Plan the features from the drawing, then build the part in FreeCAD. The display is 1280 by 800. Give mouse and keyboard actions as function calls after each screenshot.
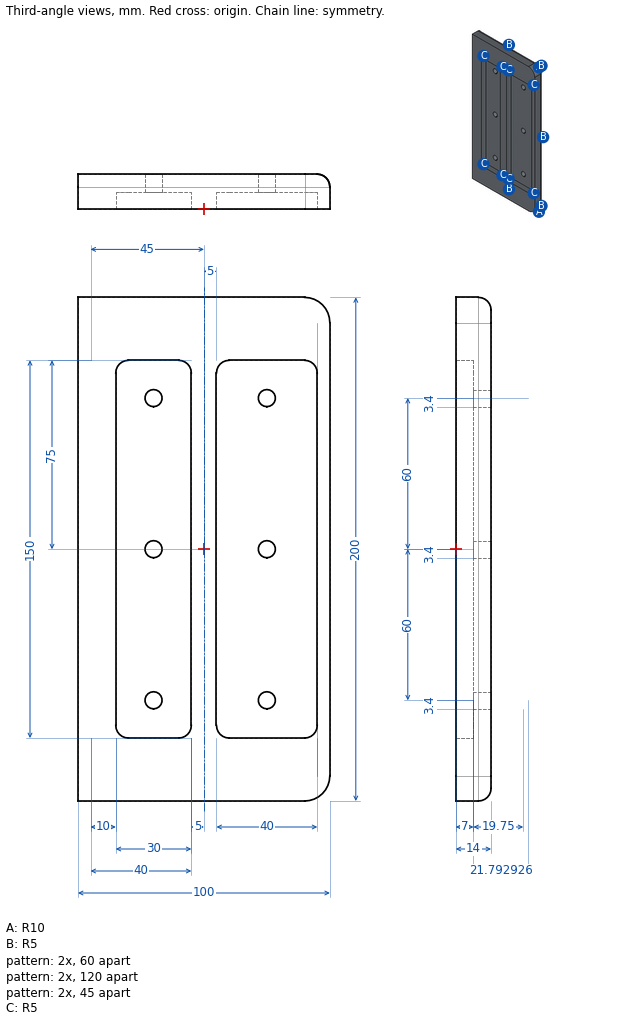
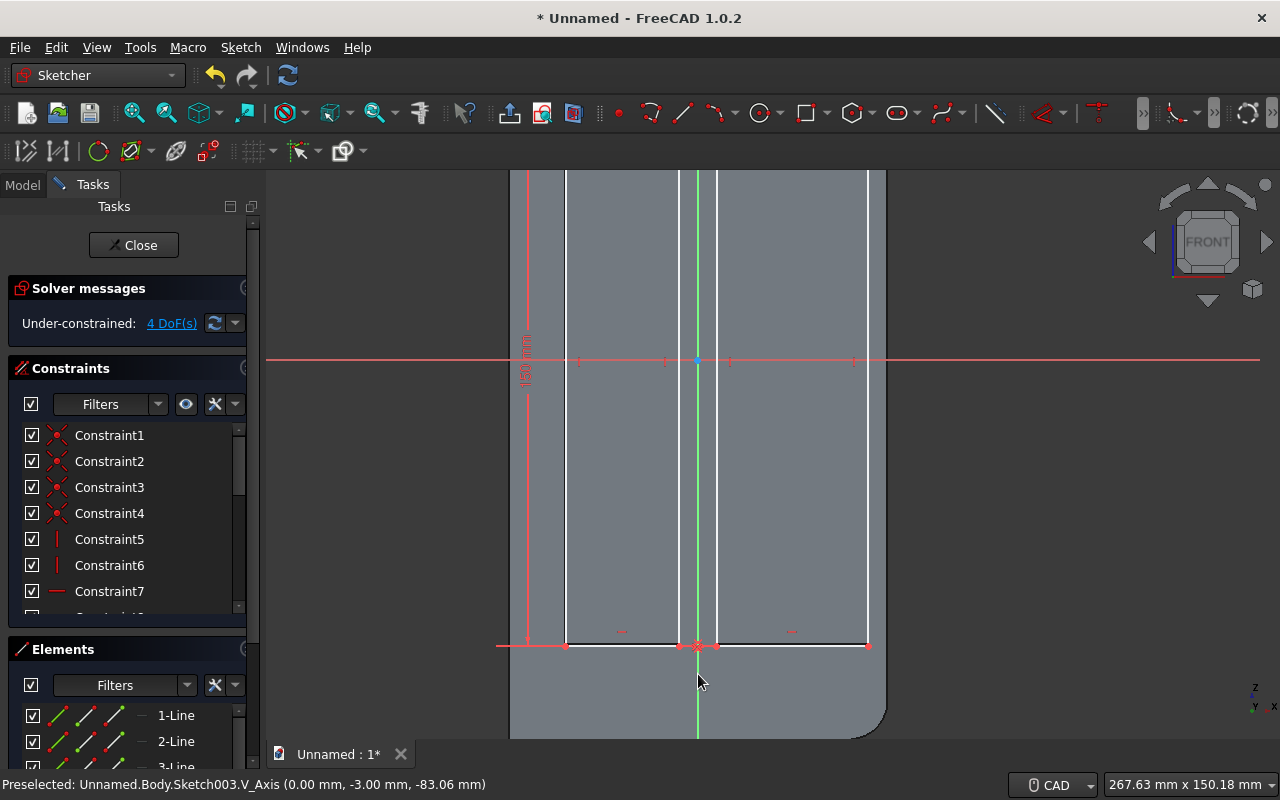
click(1042, 114)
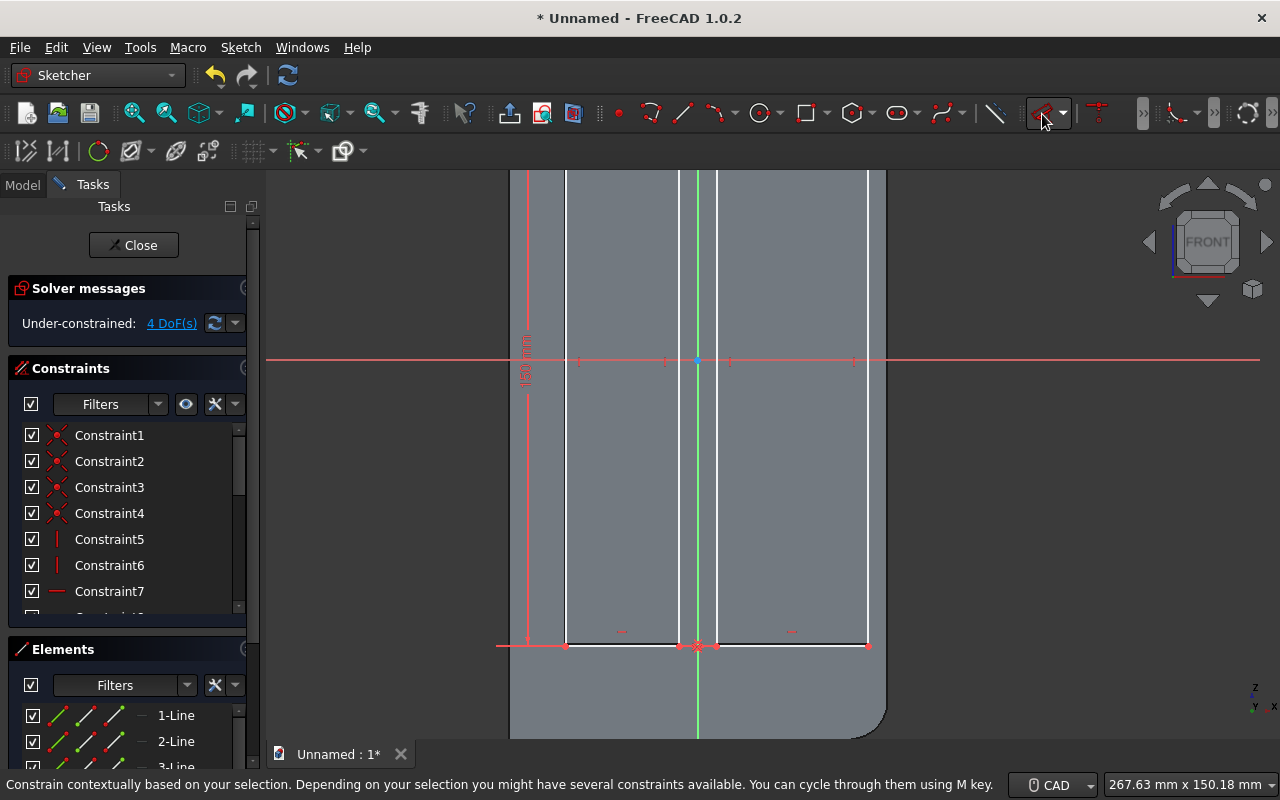
click(762, 646)
click(792, 680)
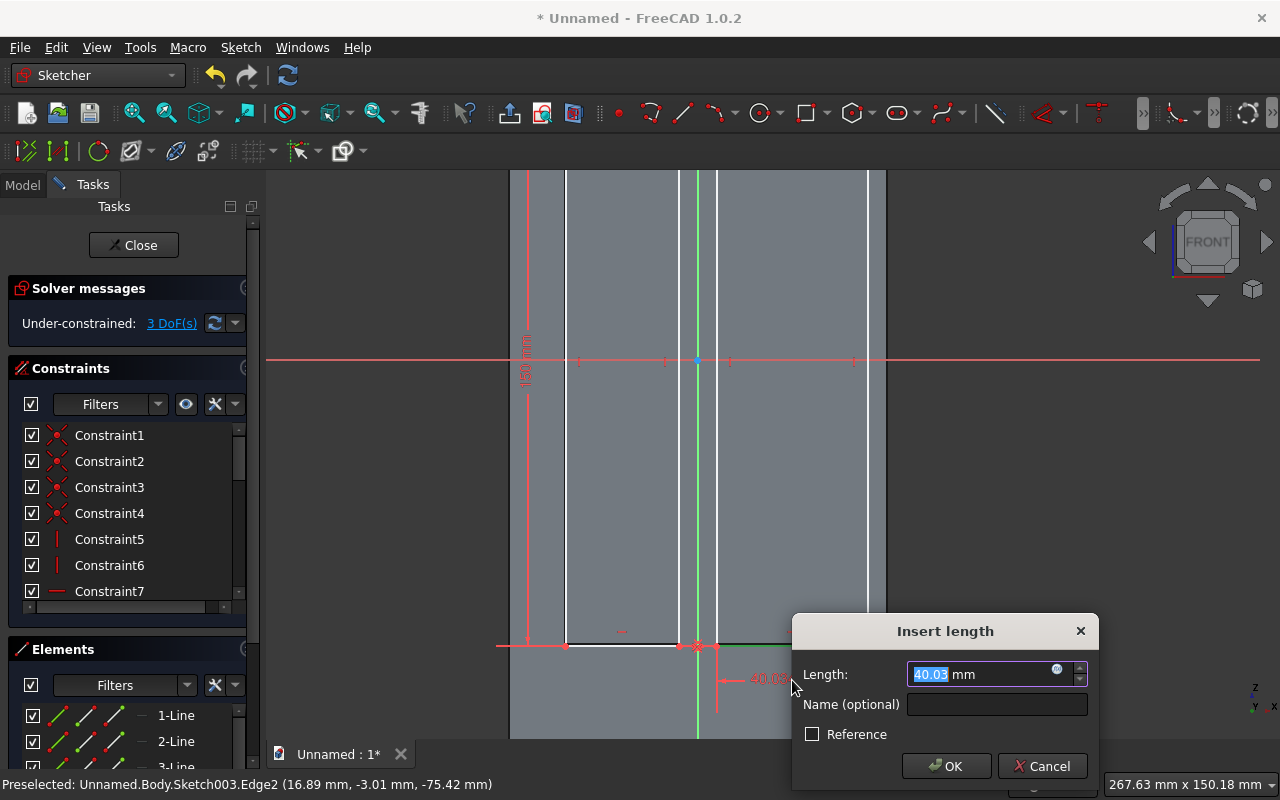
text(40)
key(Return)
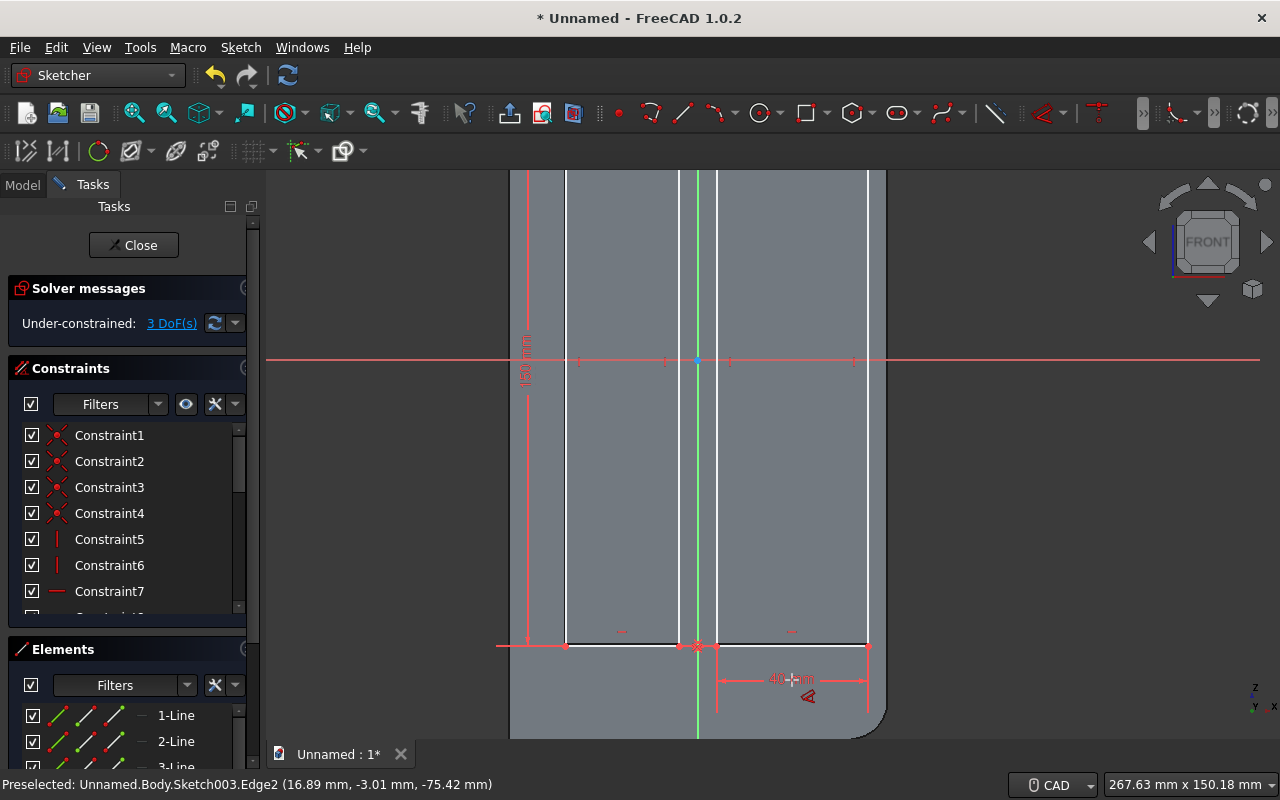
scroll(679, 646, down, 2)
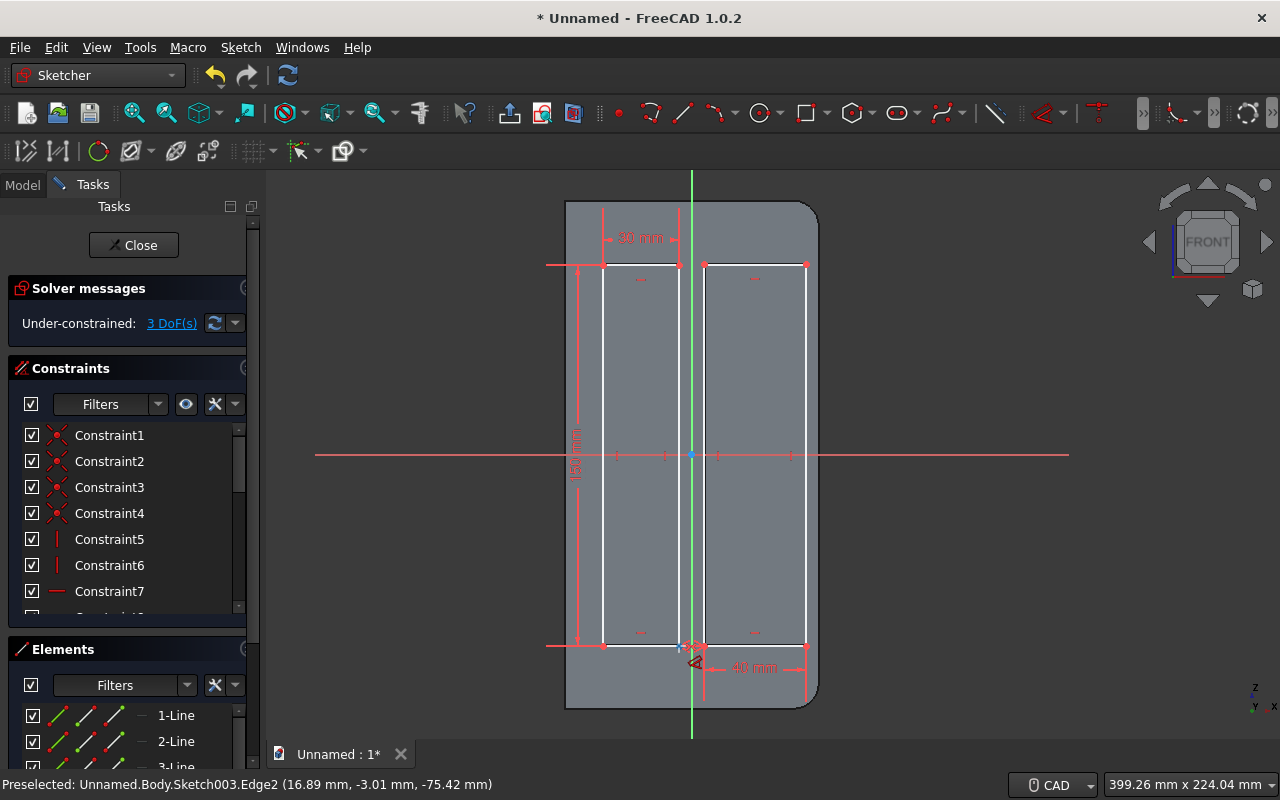
scroll(704, 265, up, 6)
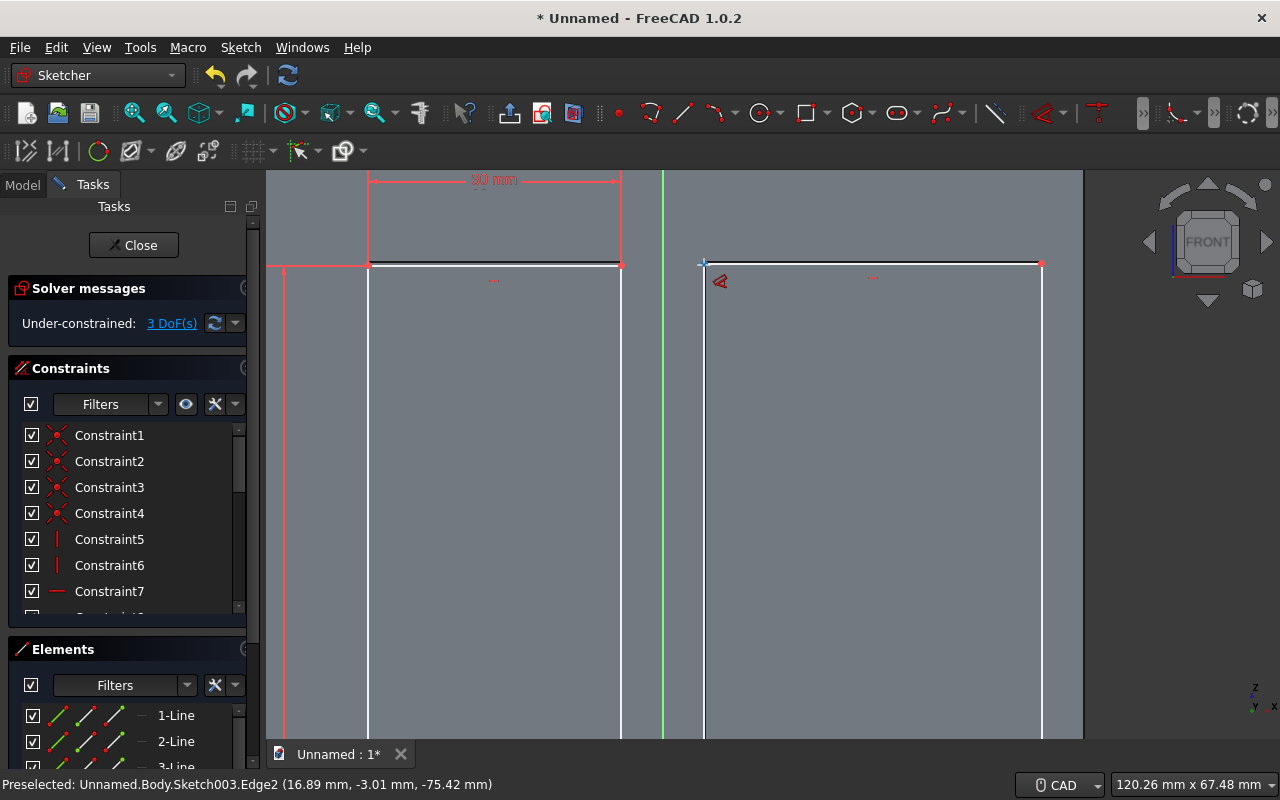
click(704, 264)
click(684, 230)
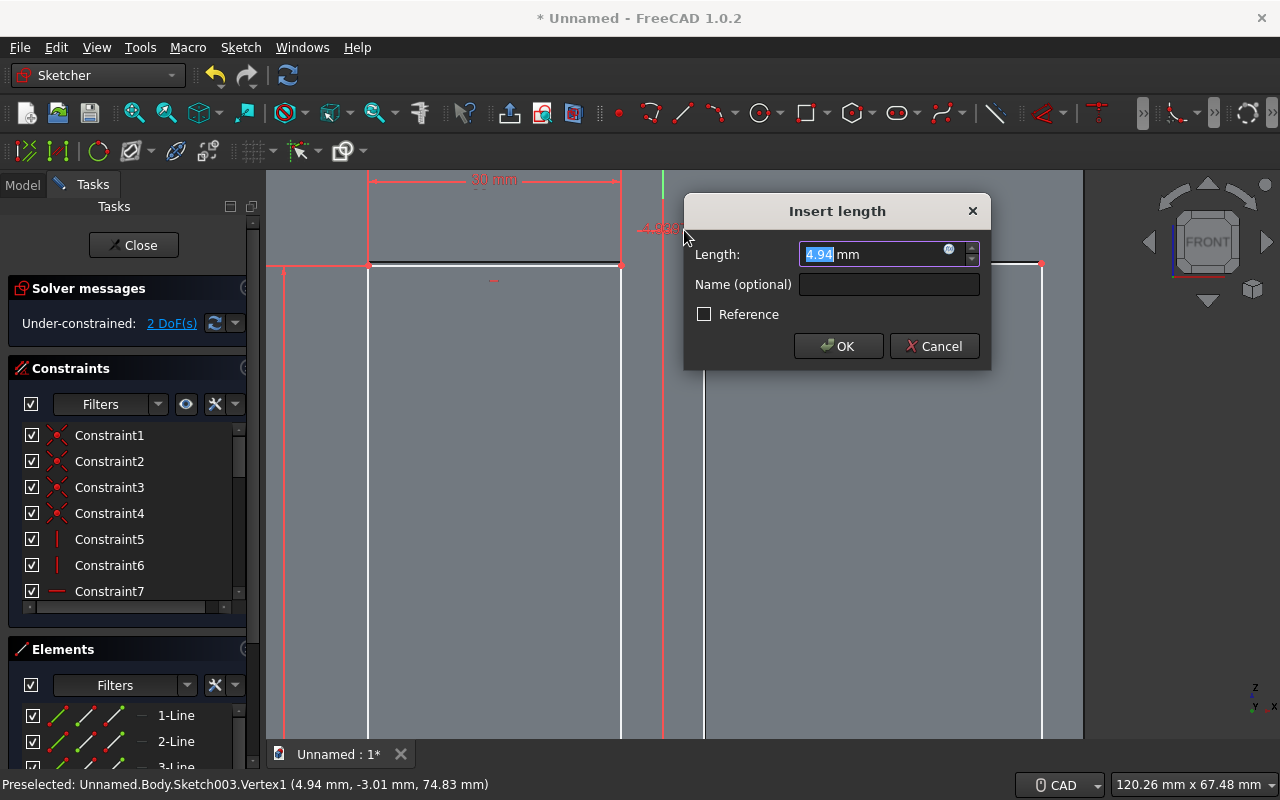
text(5)
key(Return)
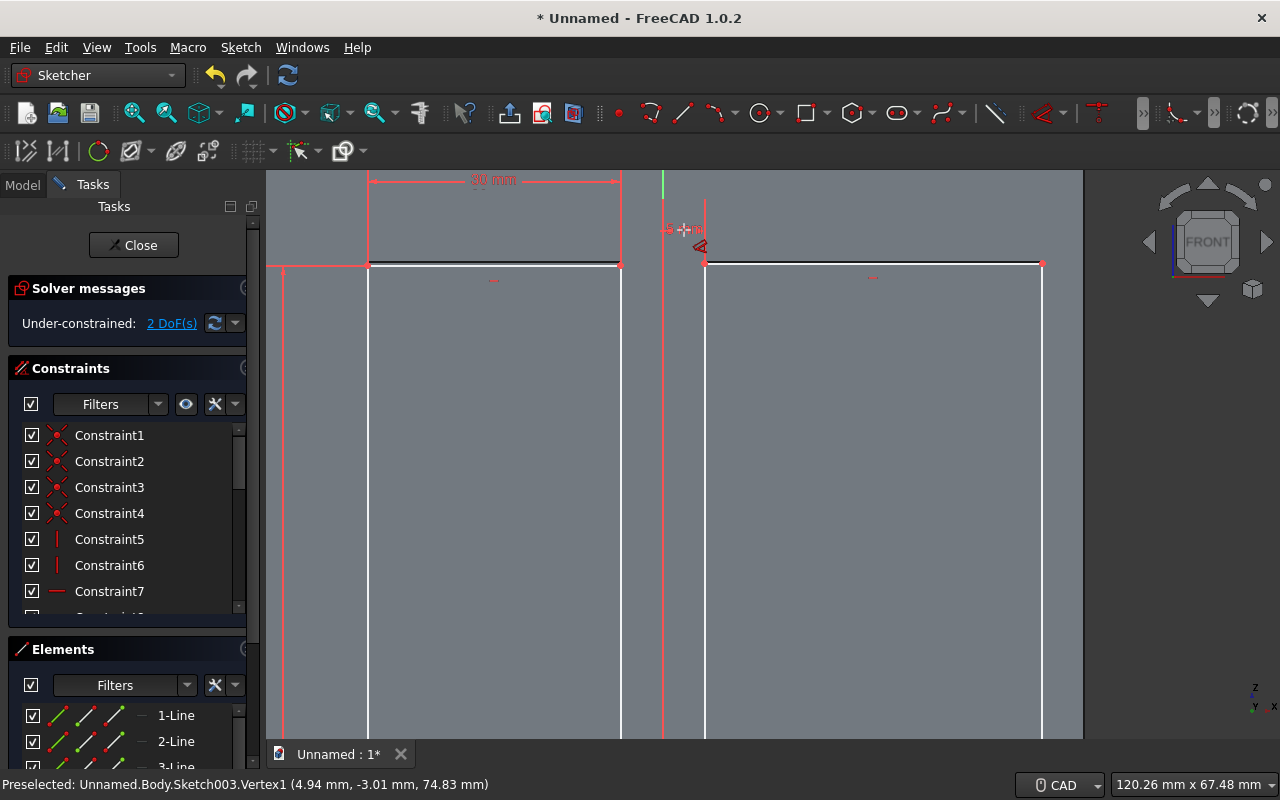
click(705, 644)
click(739, 487)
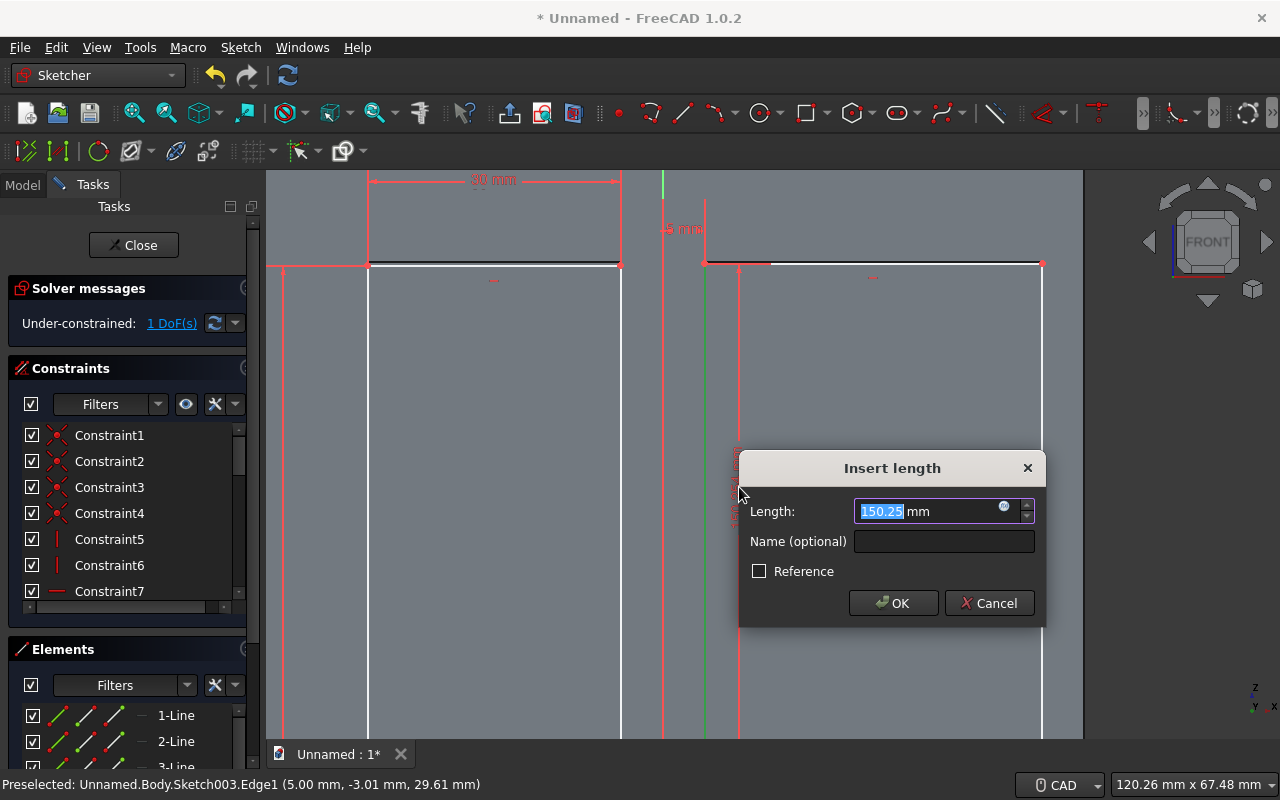
text(150)
key(Return)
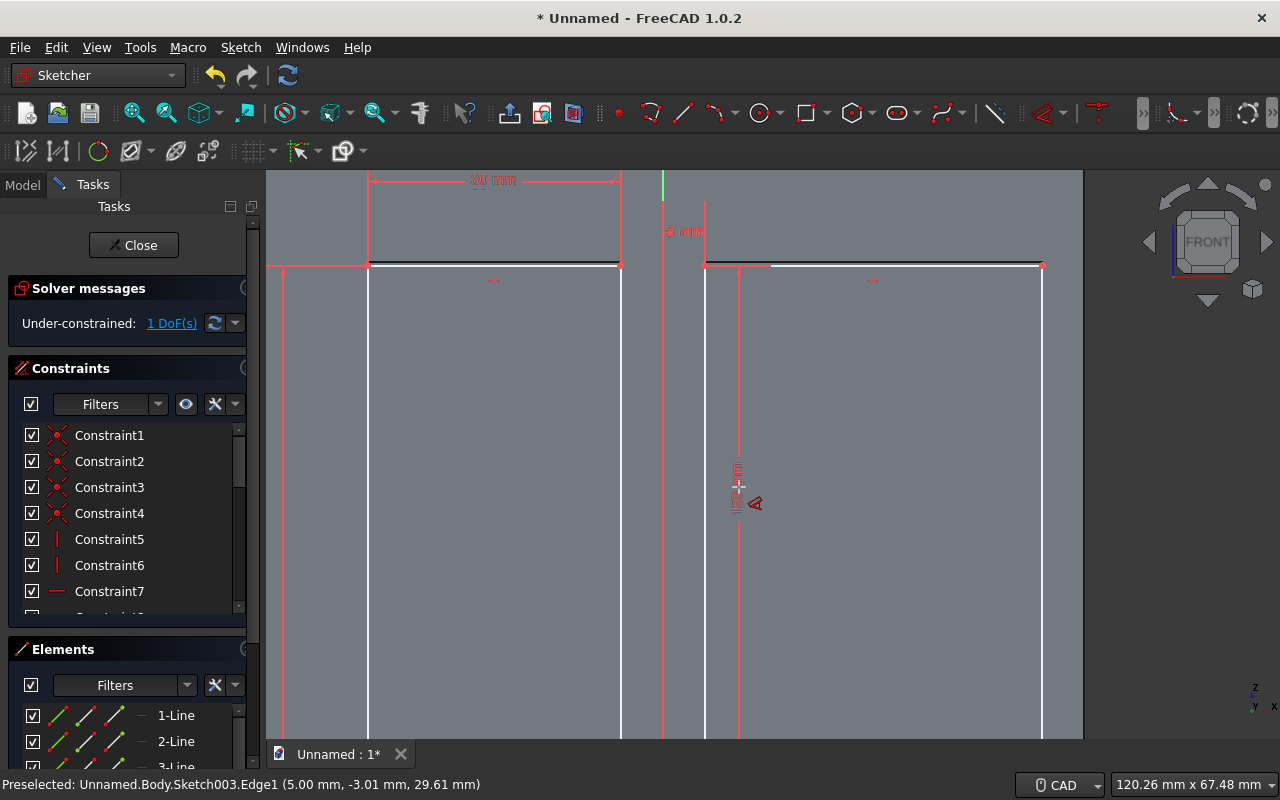
click(705, 266)
click(739, 386)